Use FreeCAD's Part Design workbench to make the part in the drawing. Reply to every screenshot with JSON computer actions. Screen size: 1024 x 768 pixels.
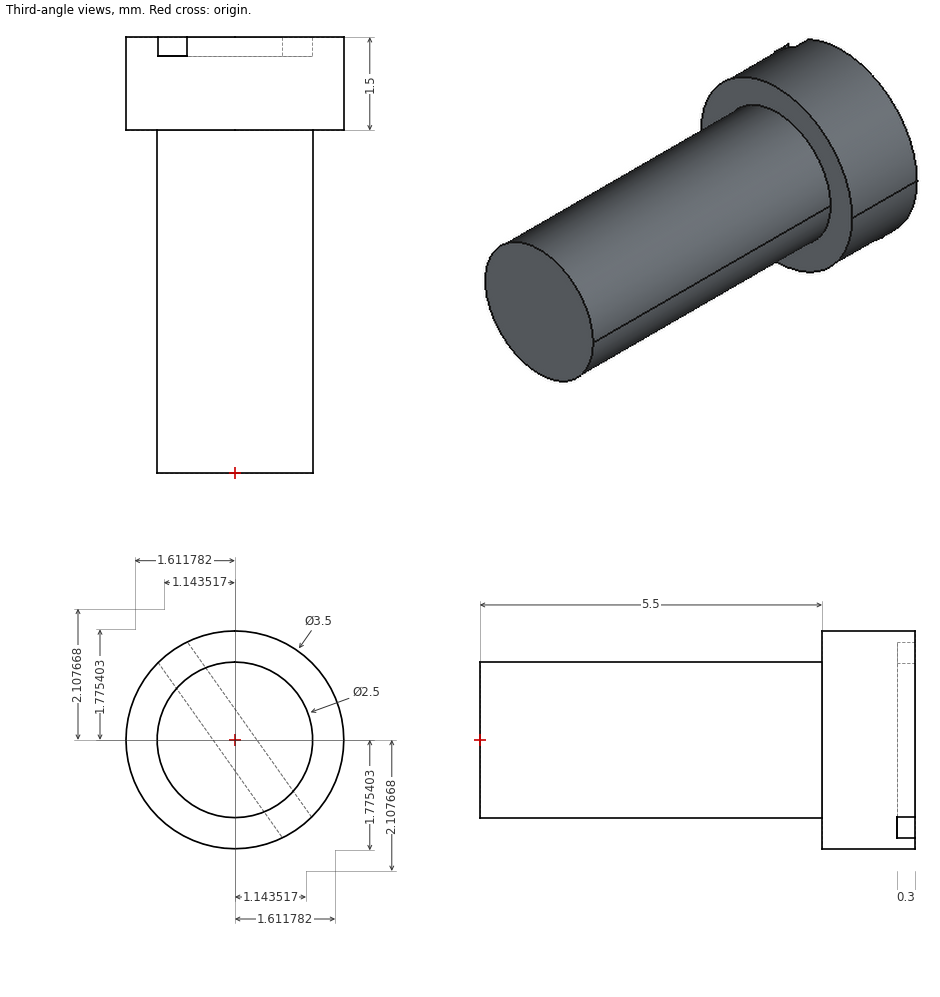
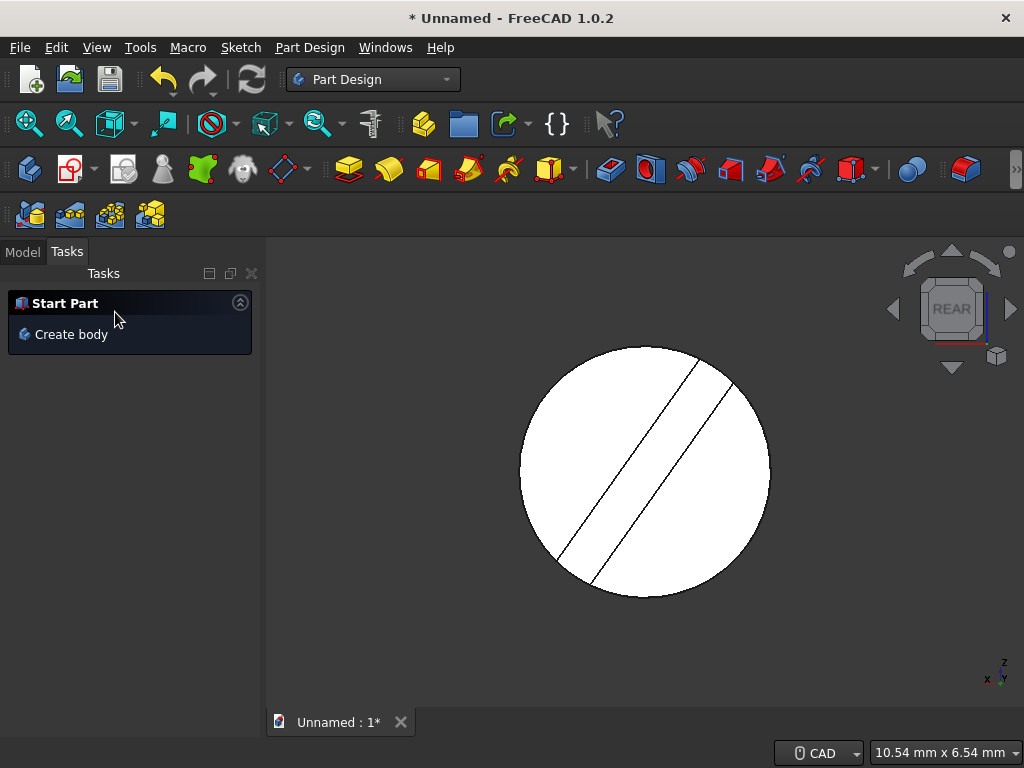
{"action": "key", "text": "0"}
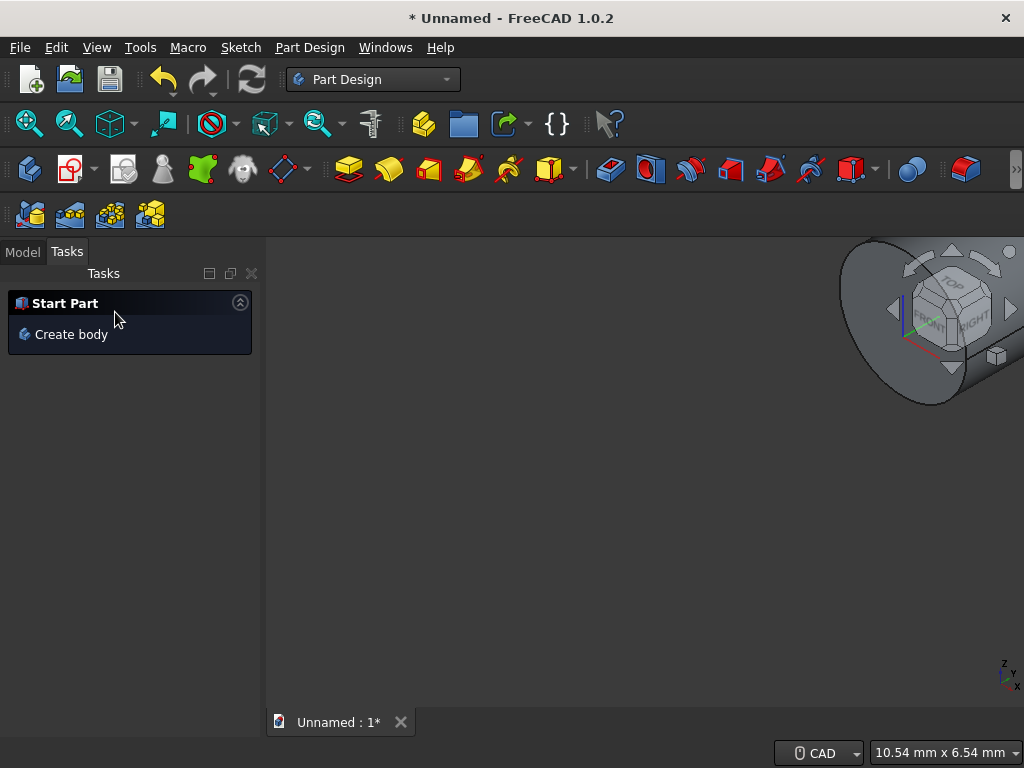
{"action": "left_click", "coordinate": [30, 124]}